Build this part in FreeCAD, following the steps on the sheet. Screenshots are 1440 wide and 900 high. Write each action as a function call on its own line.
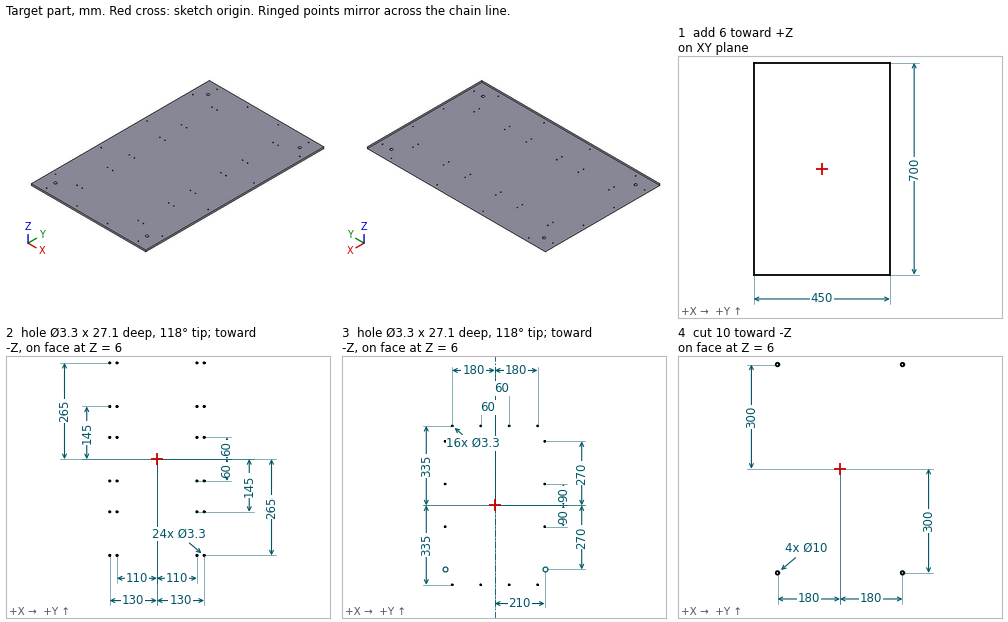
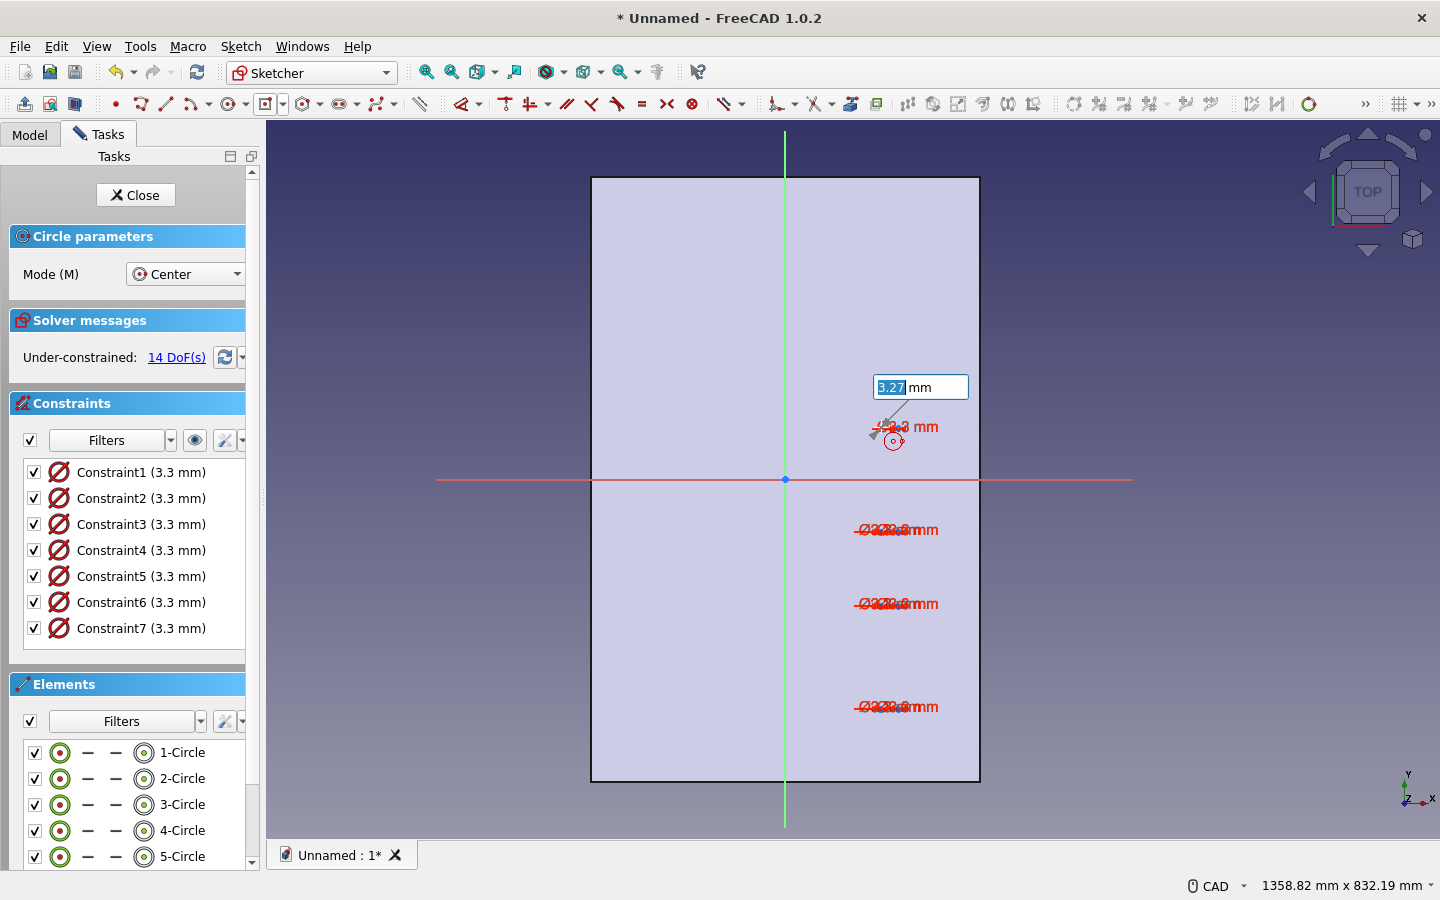
text(3.3)
key(Return)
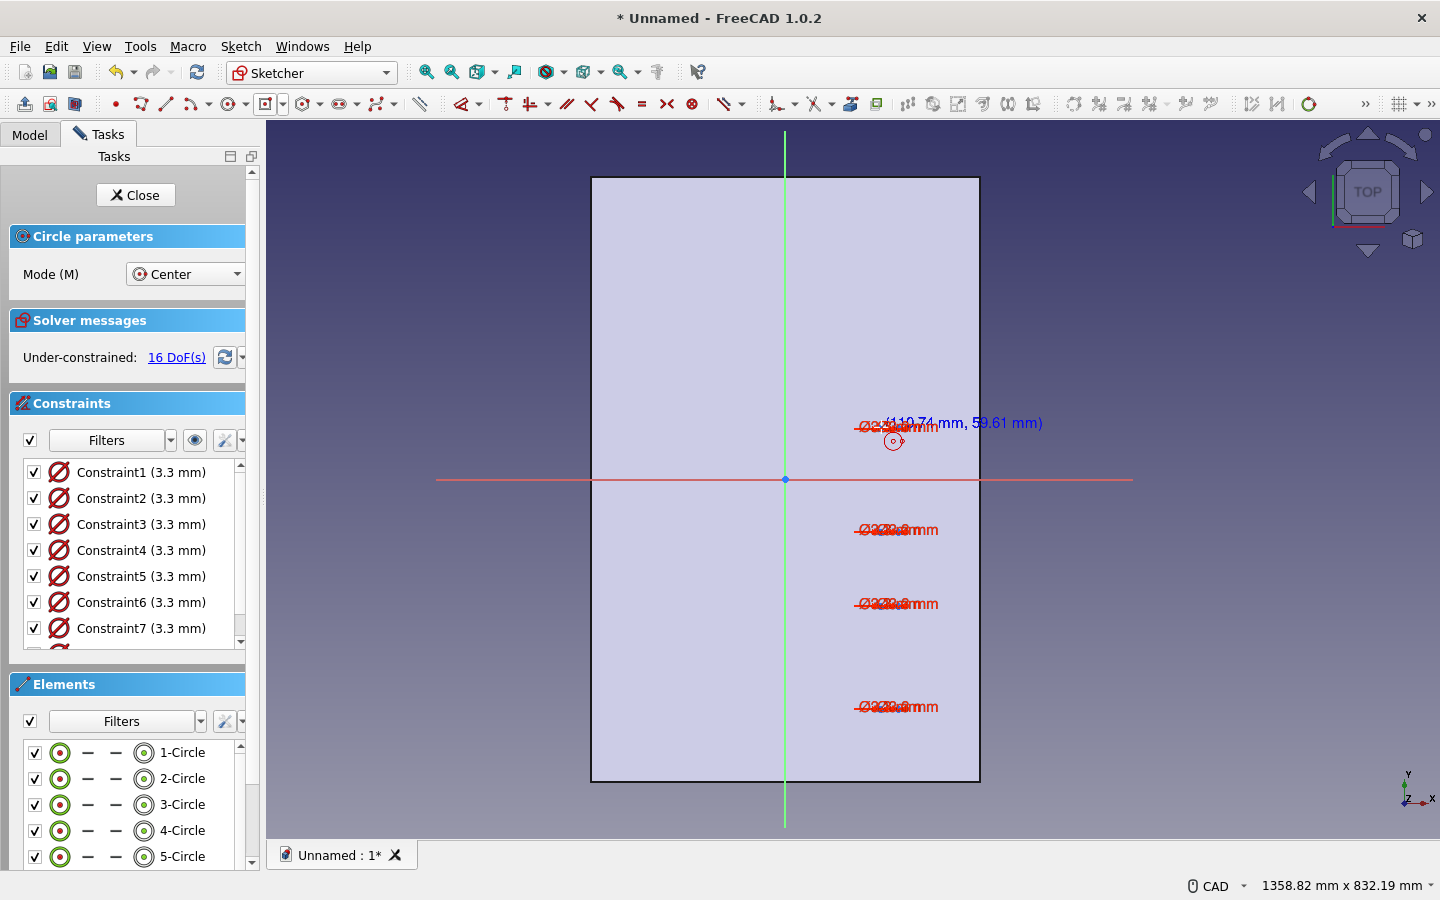
scroll(673, 708, up, 14)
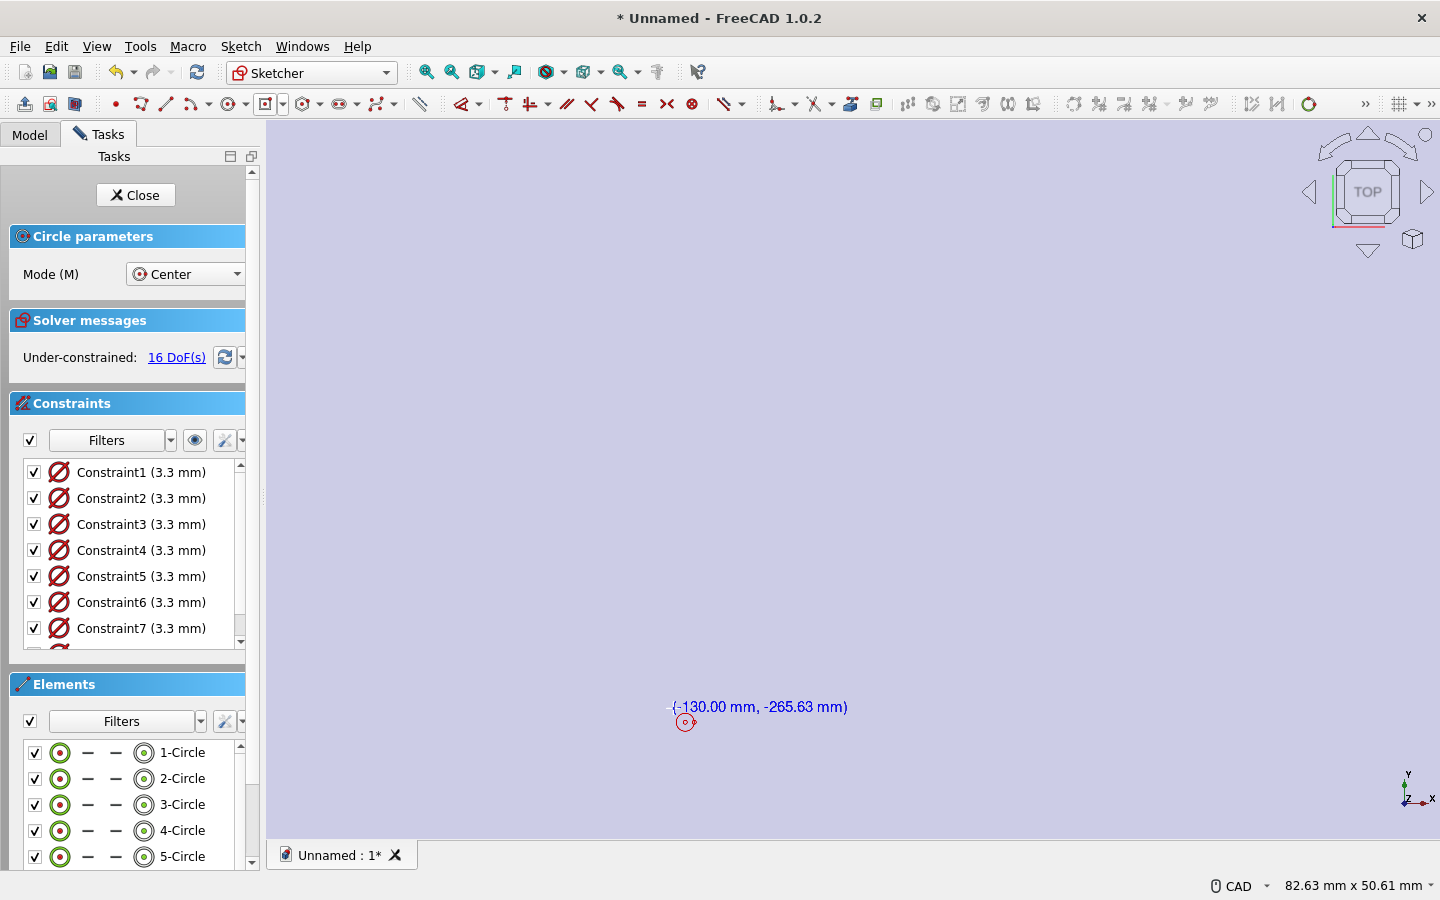
scroll(672, 709, down, 14)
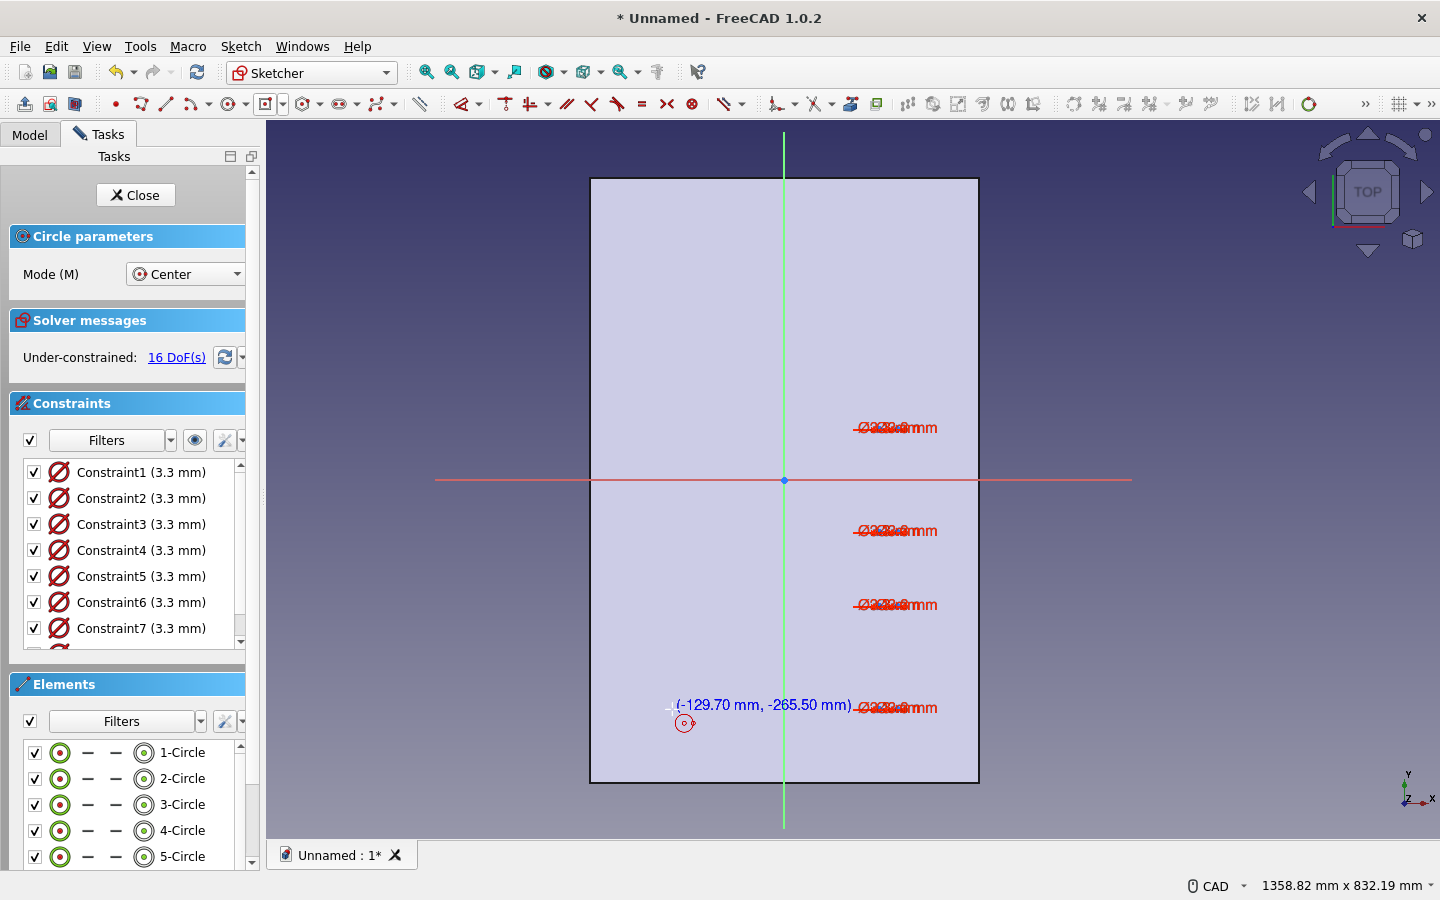
click(672, 709)
move(673, 708)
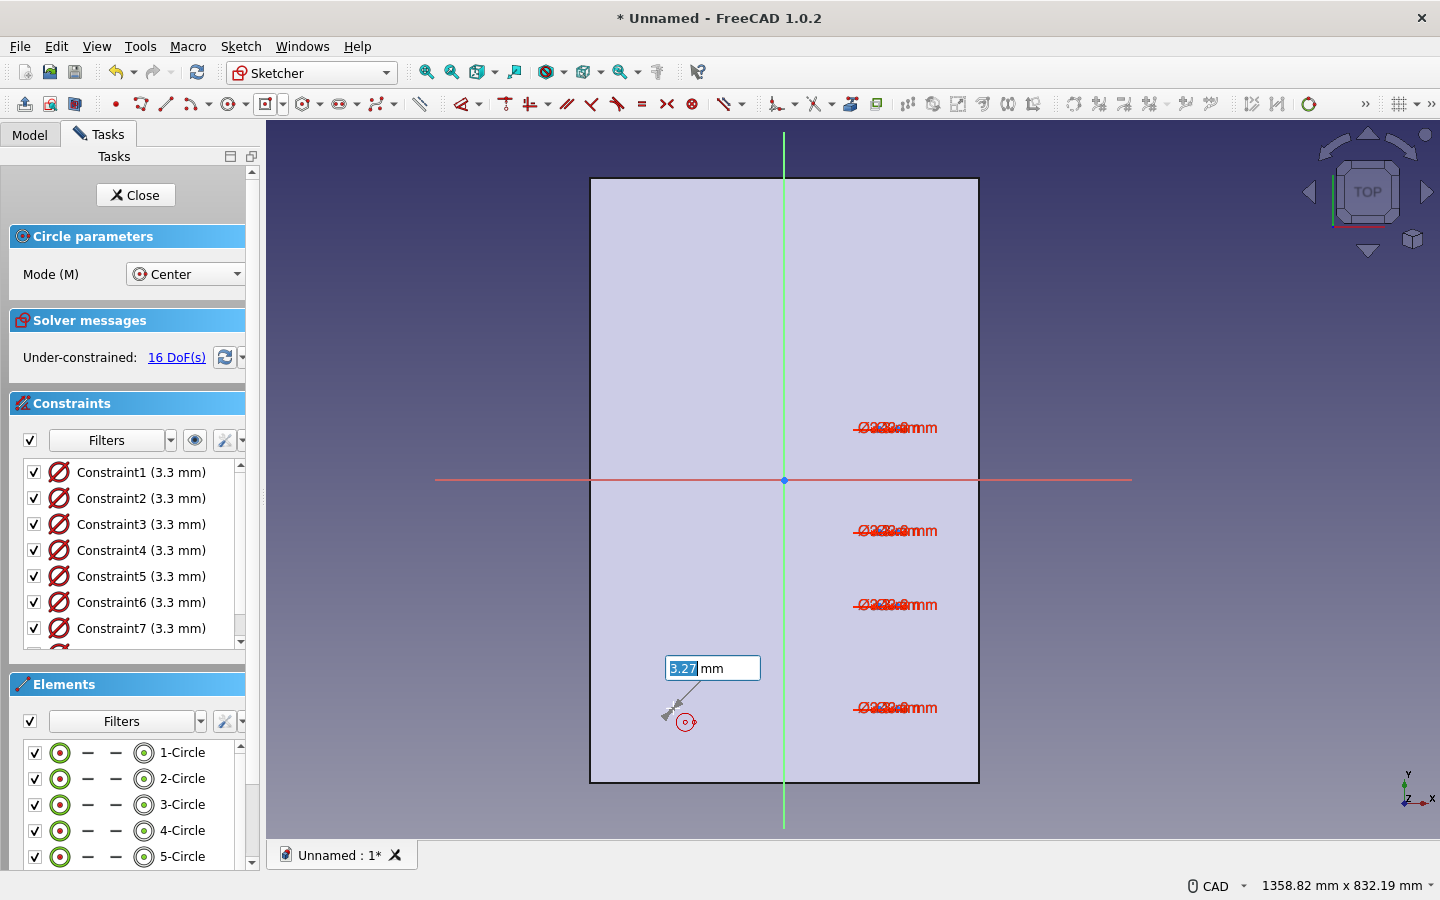
text(3.3)
key(Return)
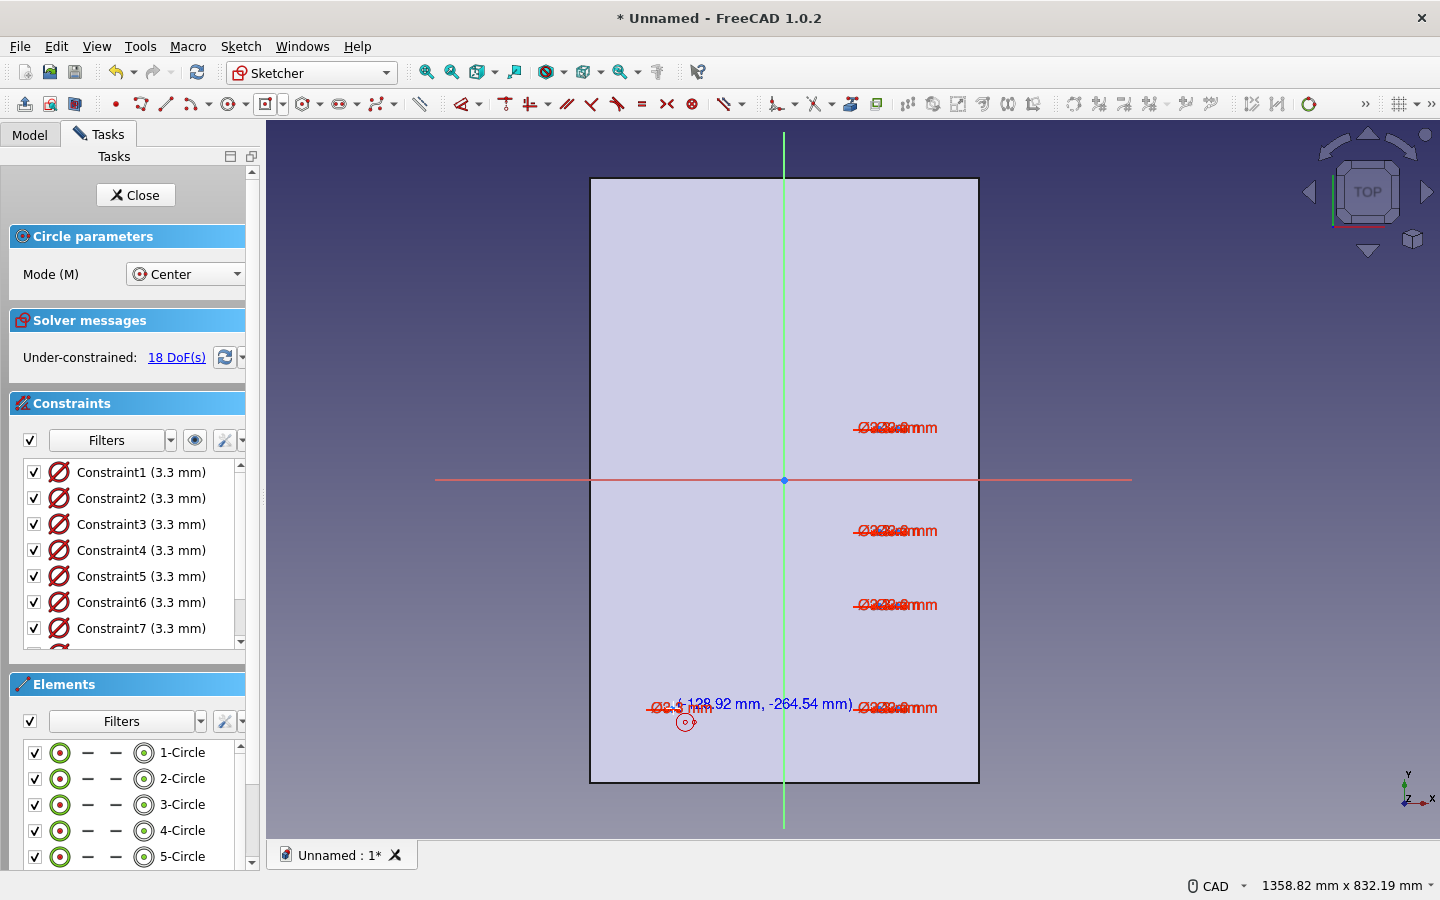
scroll(689, 709, up, 14)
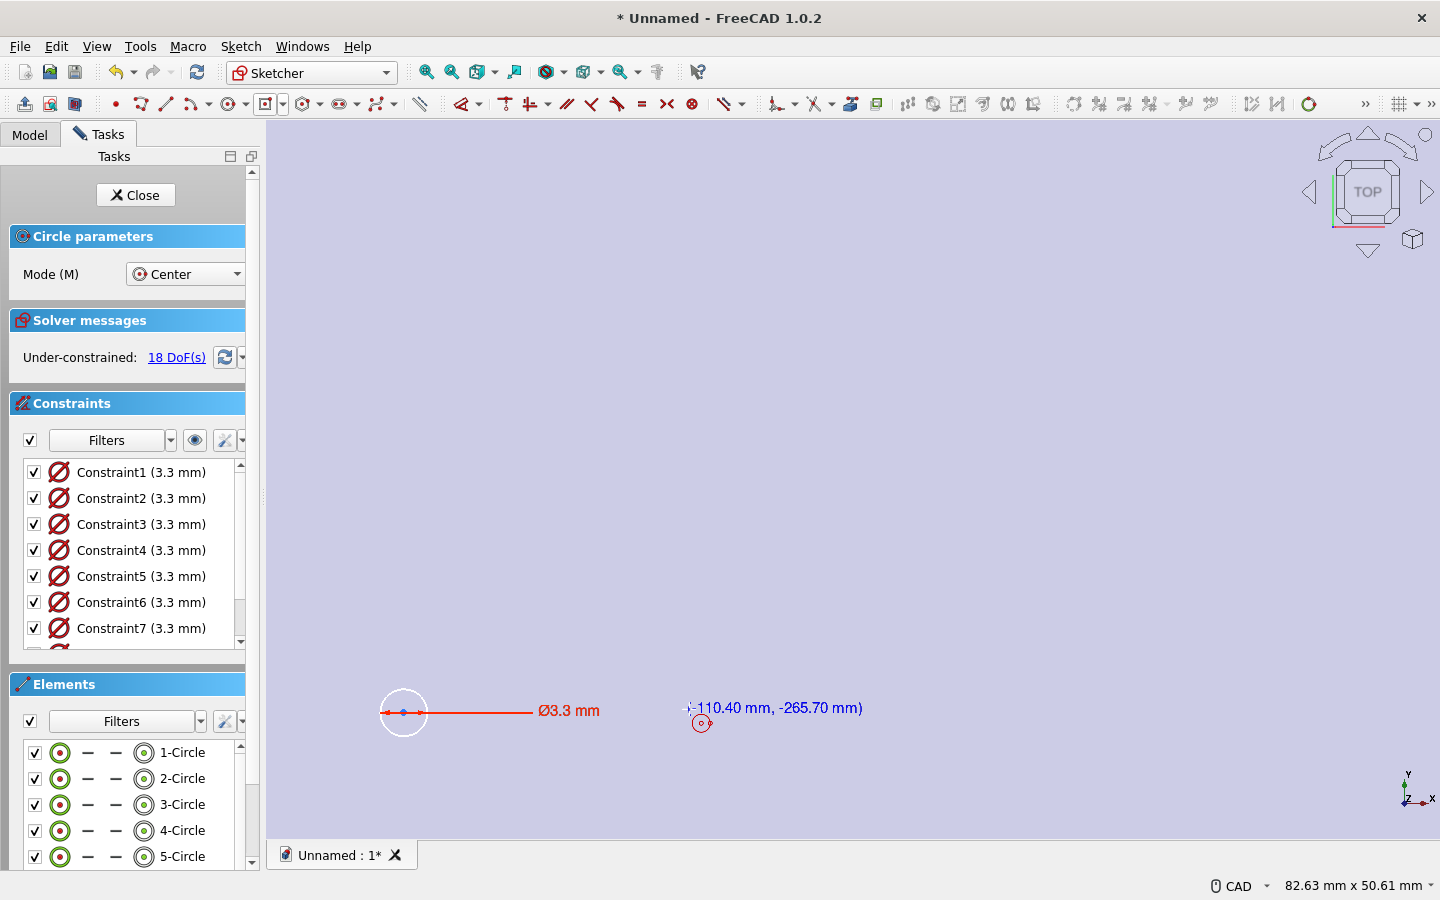
scroll(689, 709, down, 14)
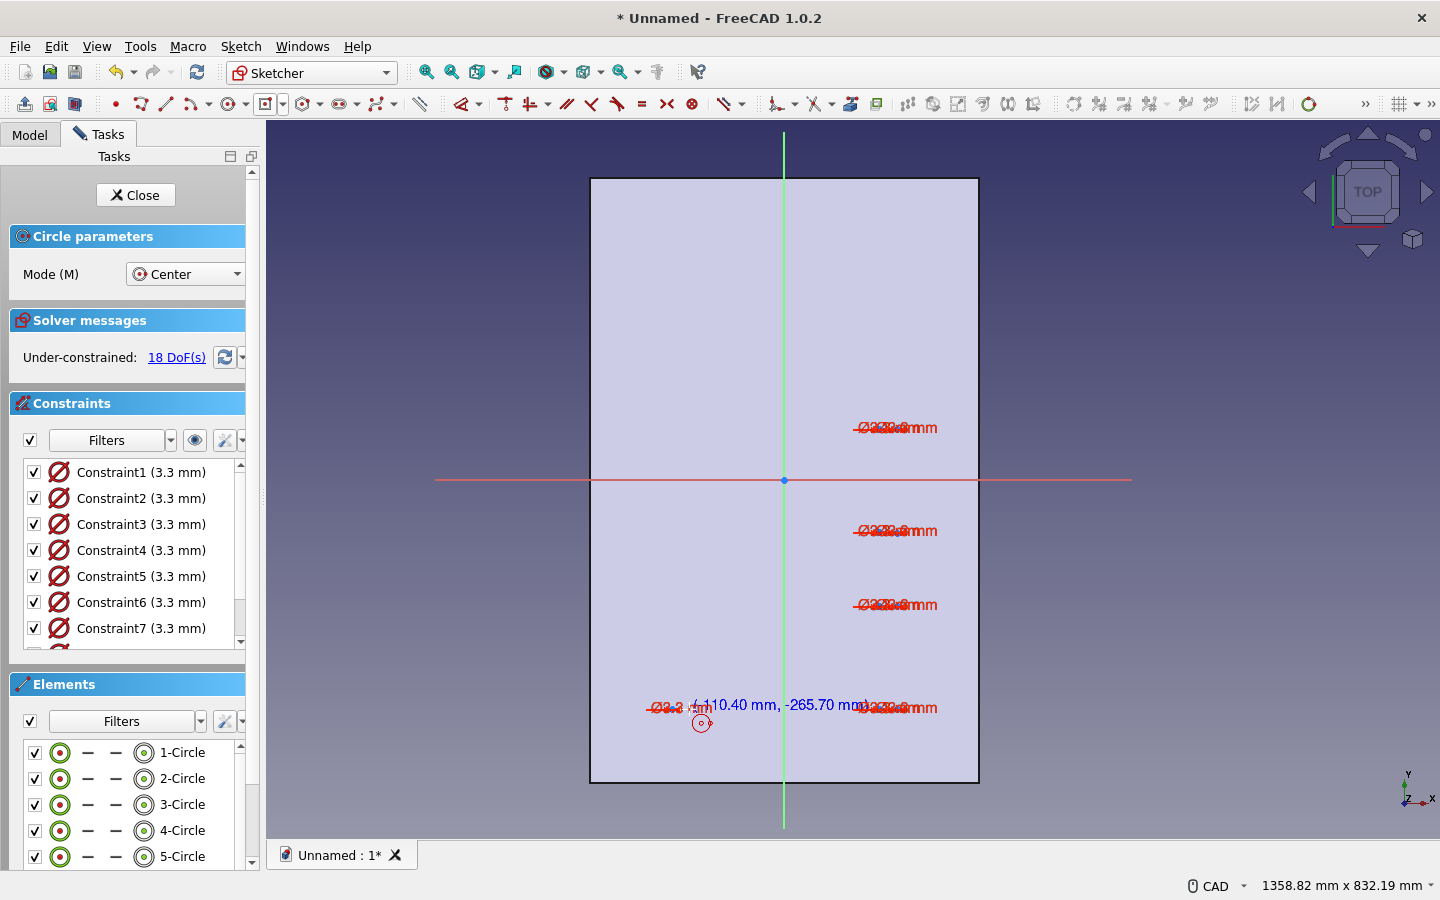
click(689, 709)
move(690, 708)